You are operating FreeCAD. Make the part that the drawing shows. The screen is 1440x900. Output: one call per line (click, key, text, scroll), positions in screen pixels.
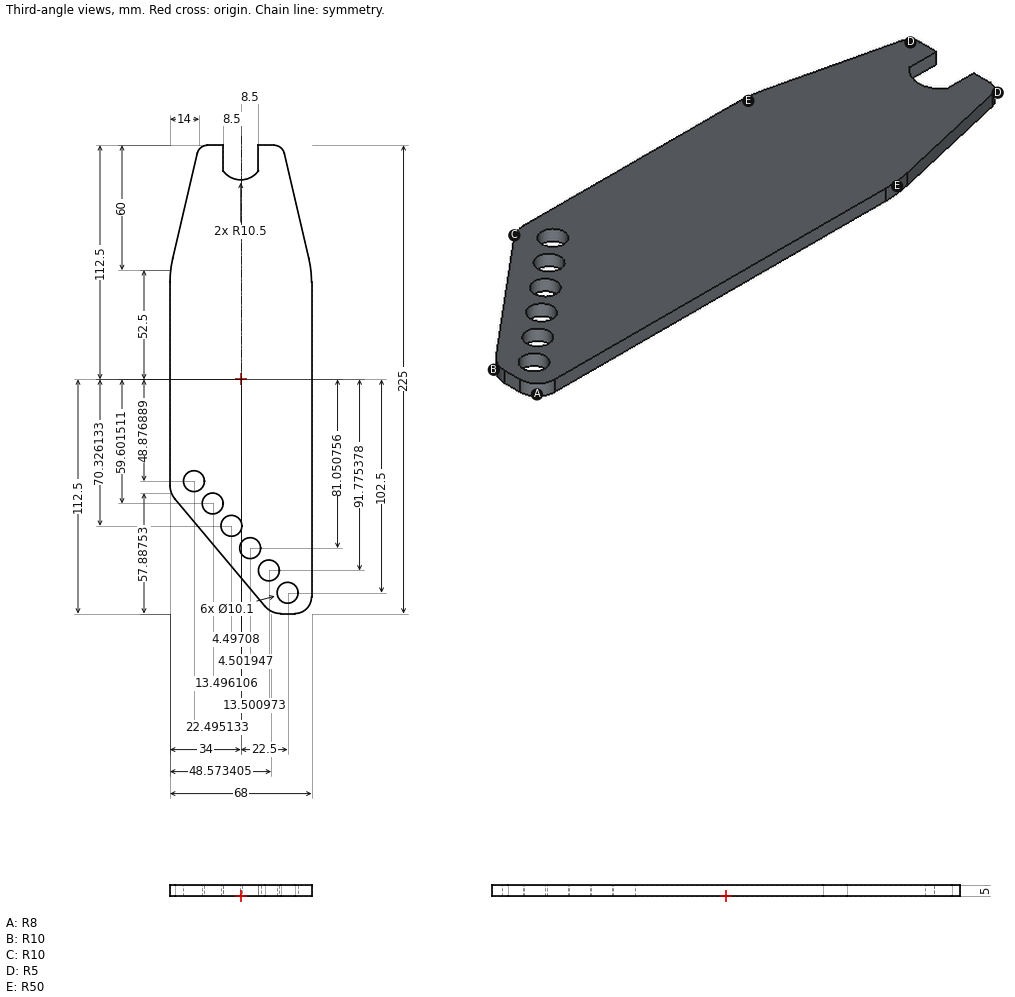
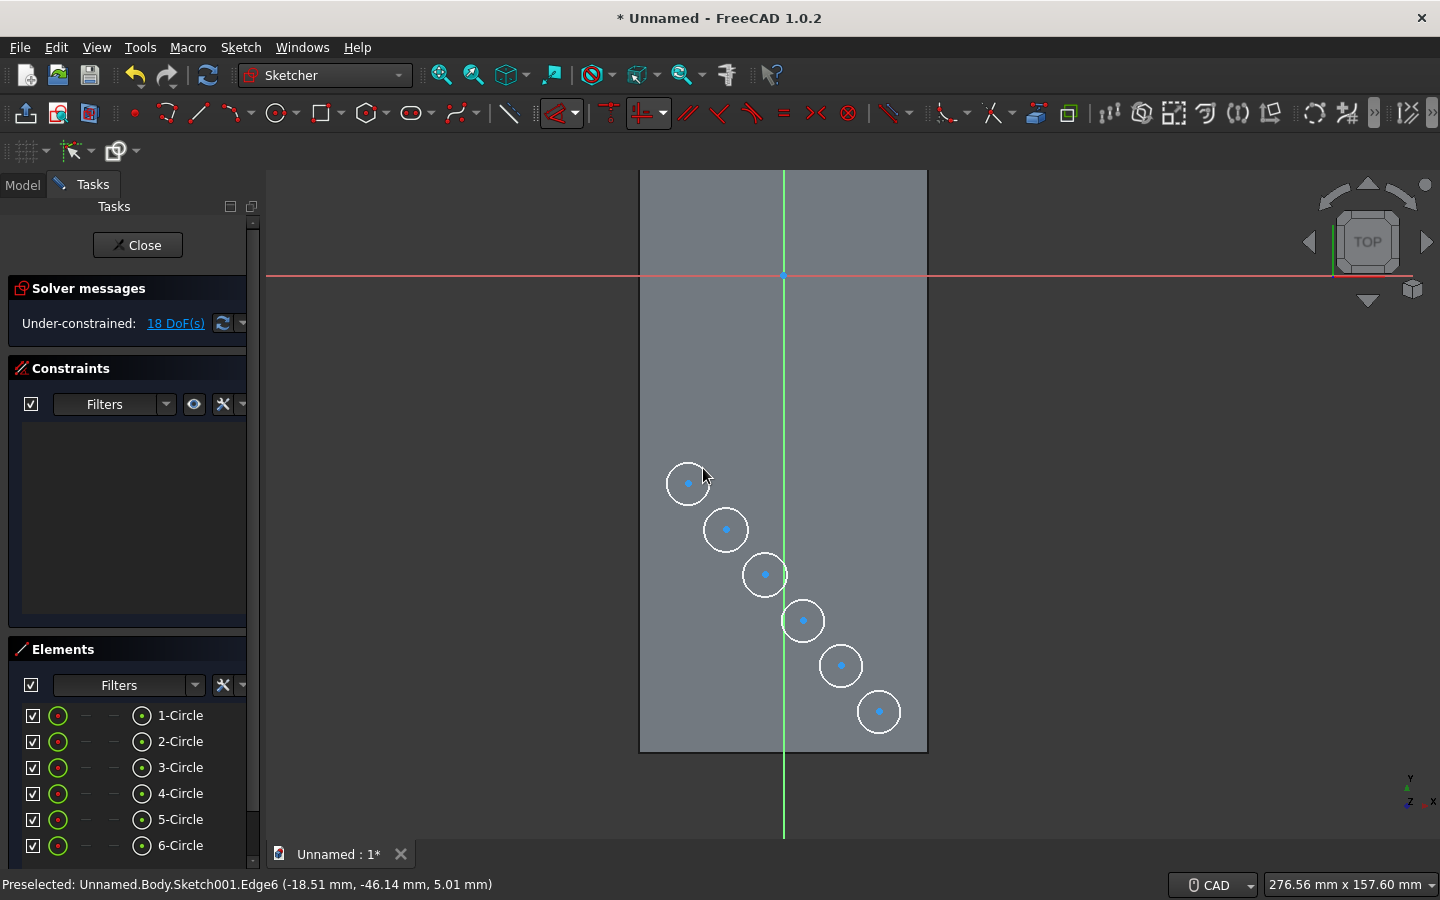
click(894, 697)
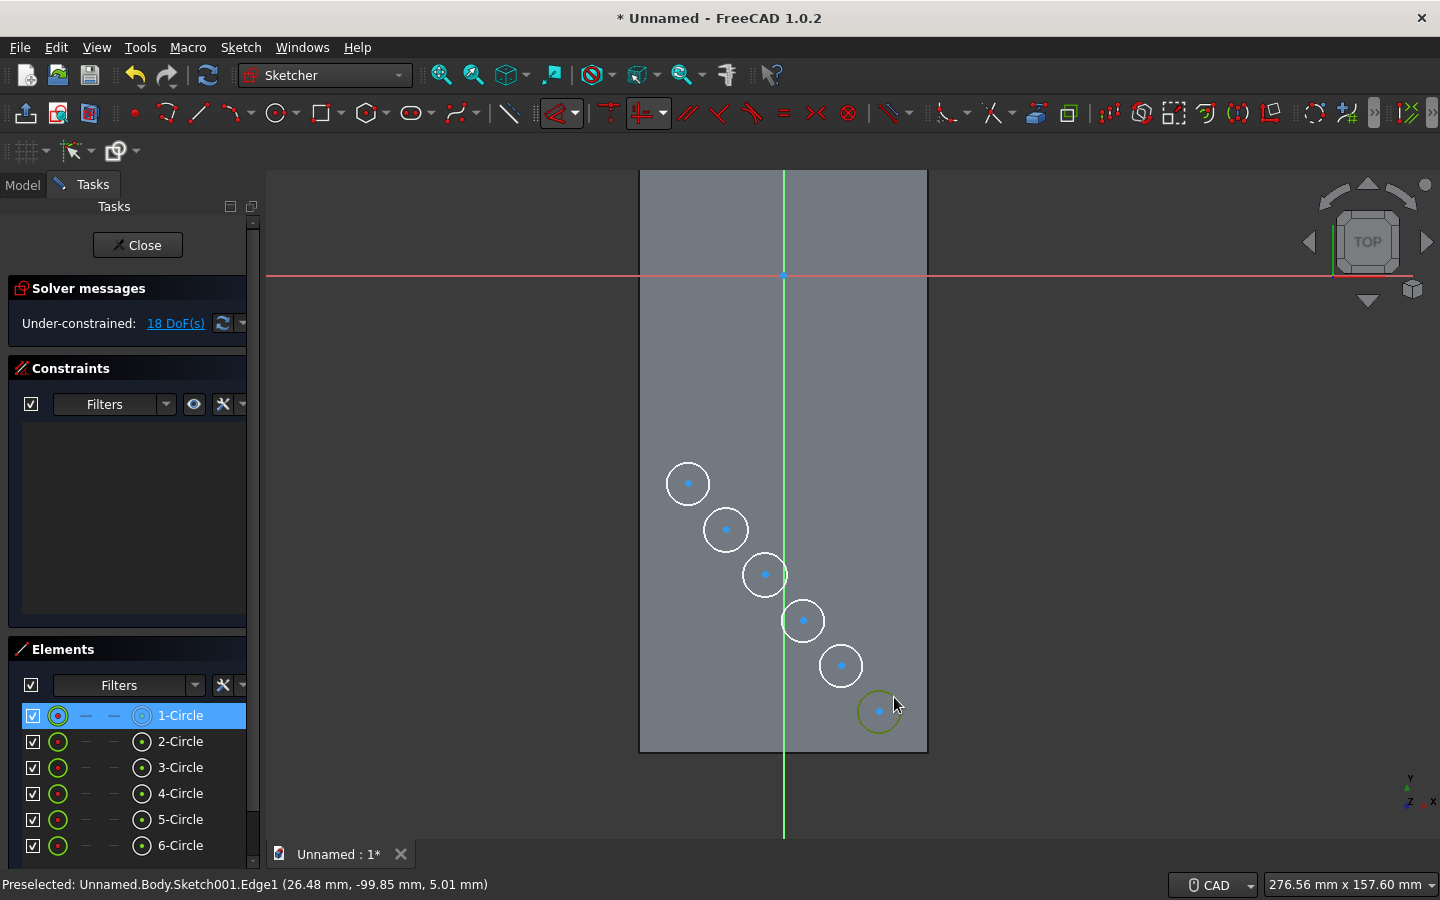
click(856, 651)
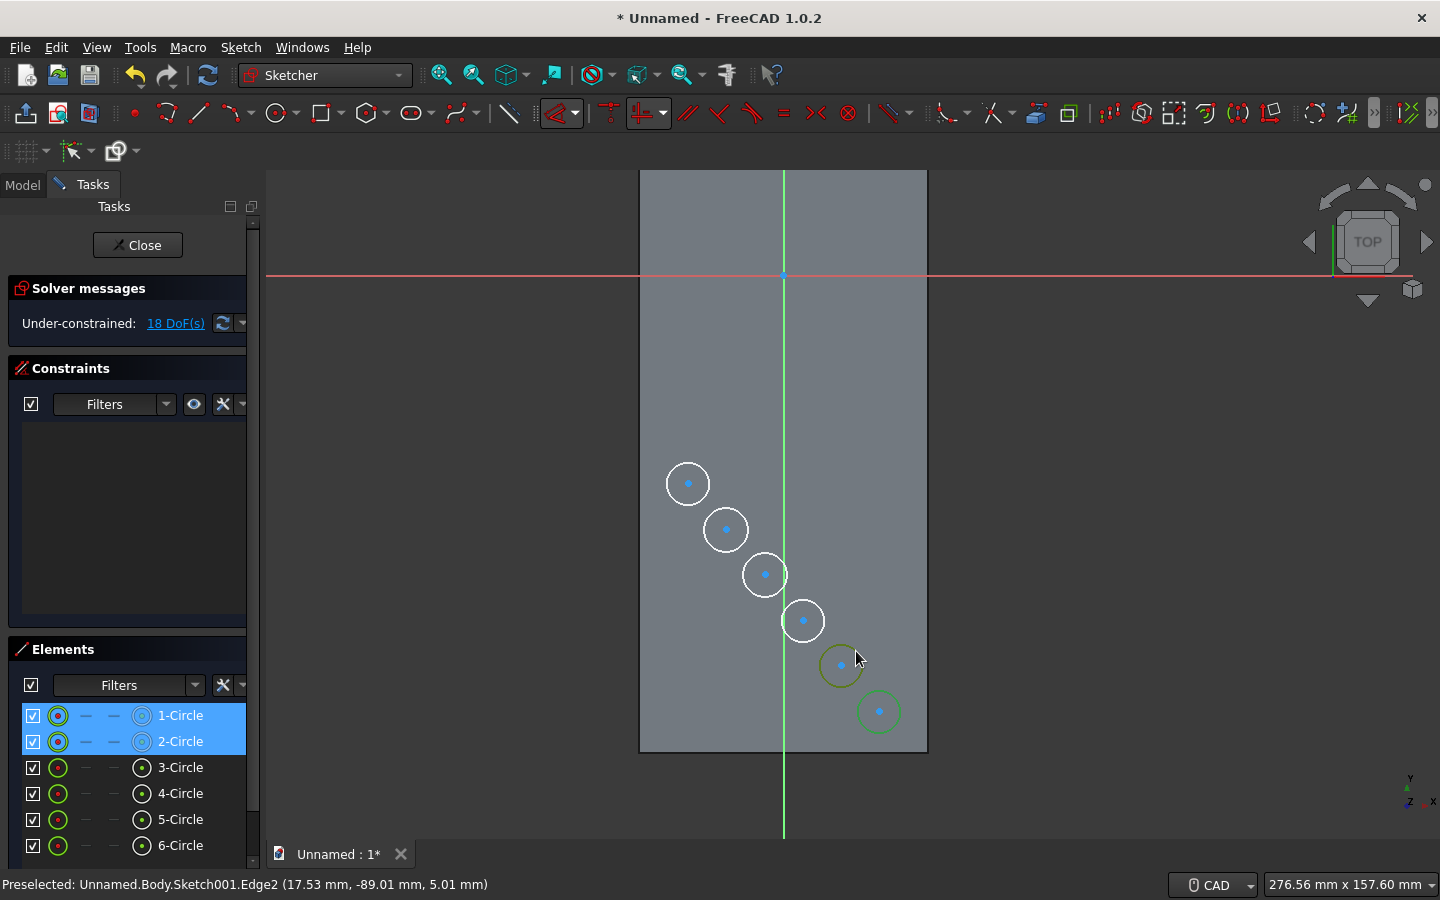
click(818, 606)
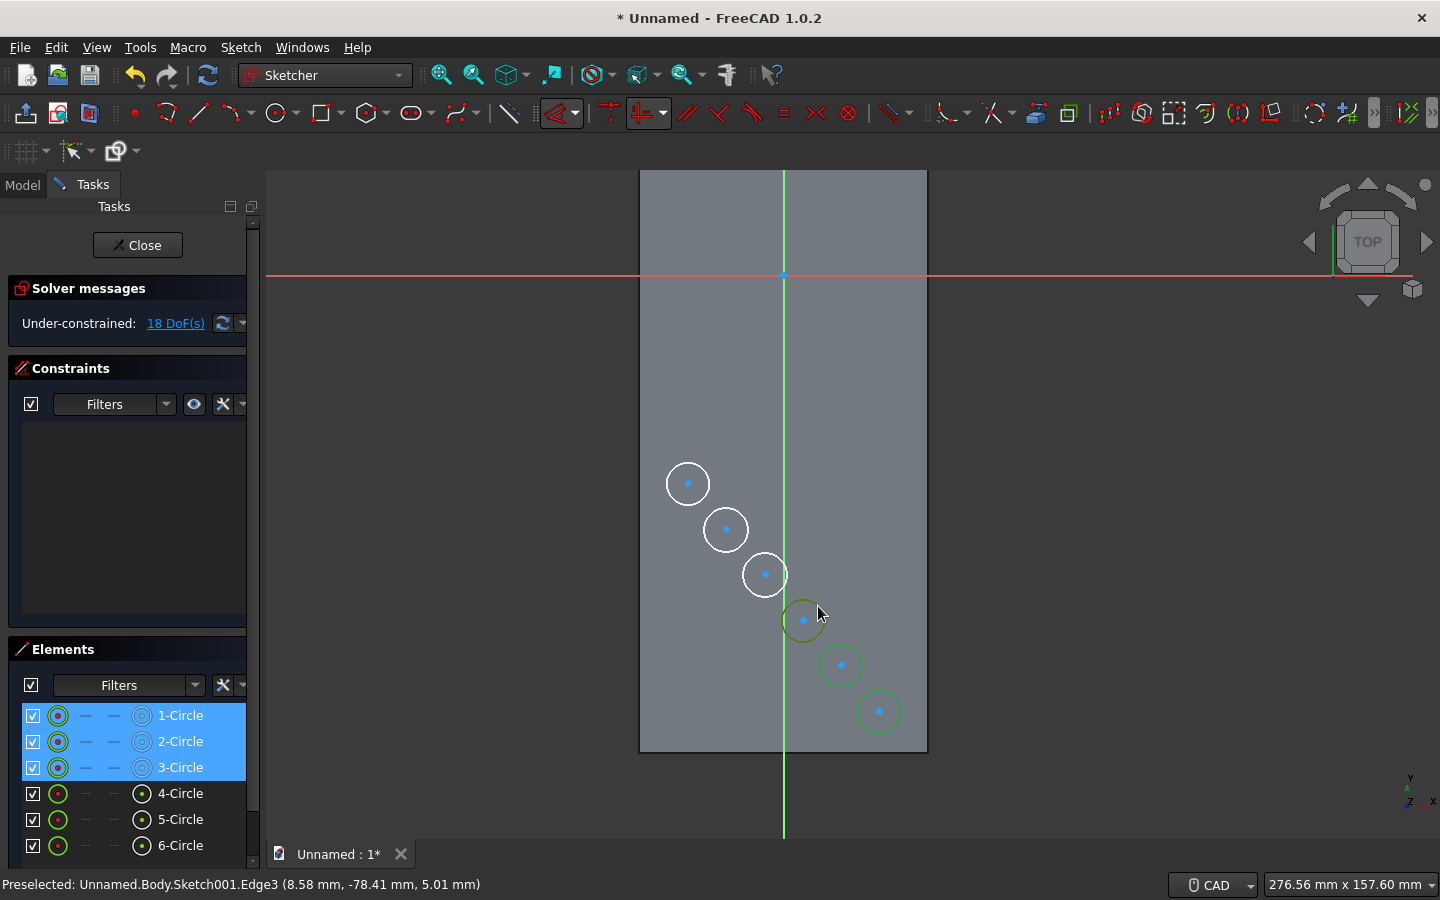
click(780, 559)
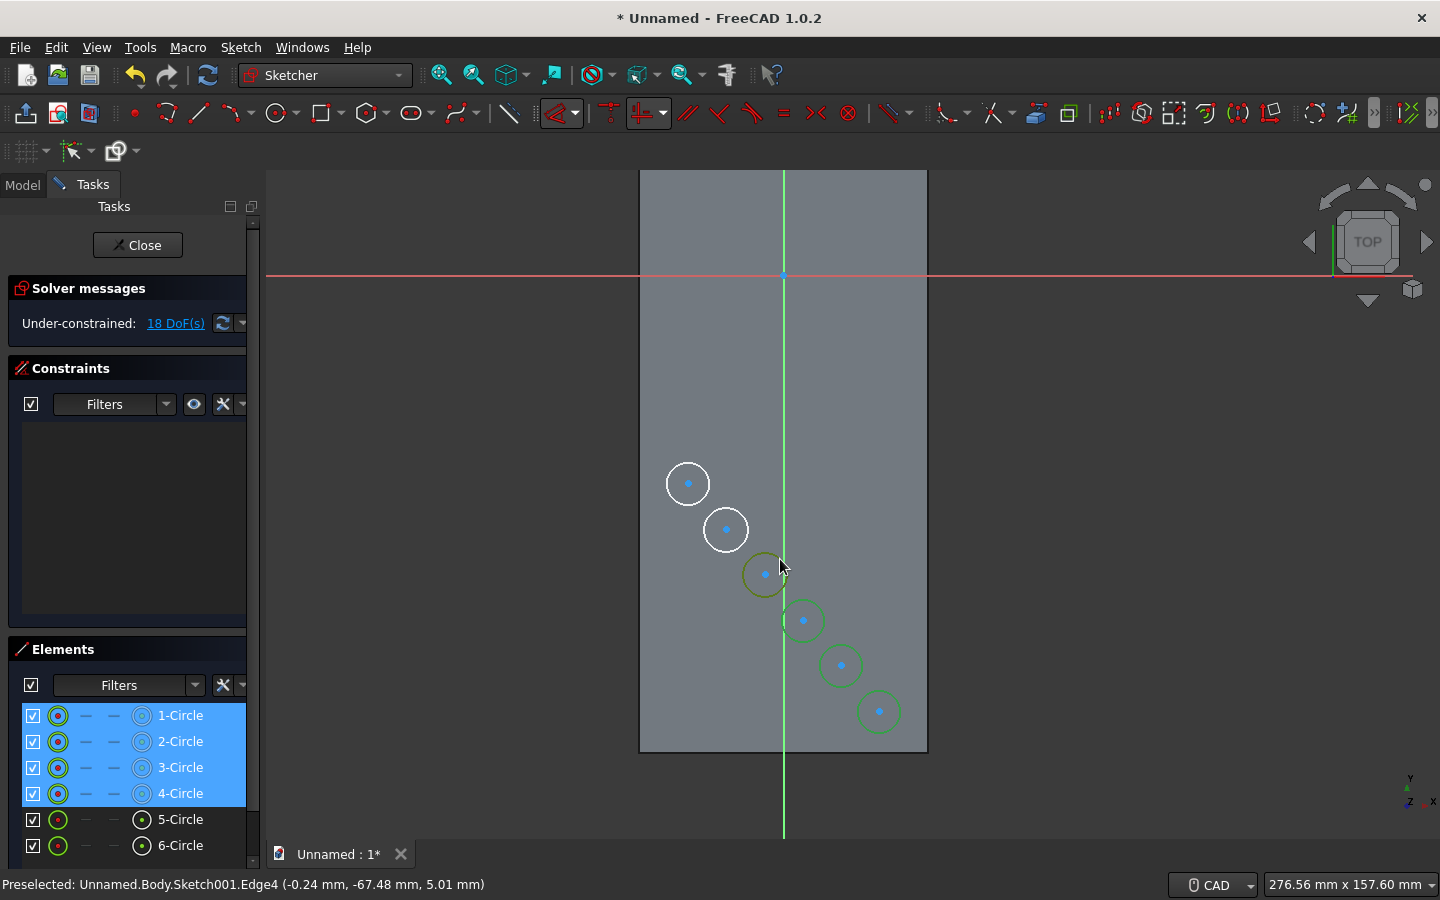
click(741, 514)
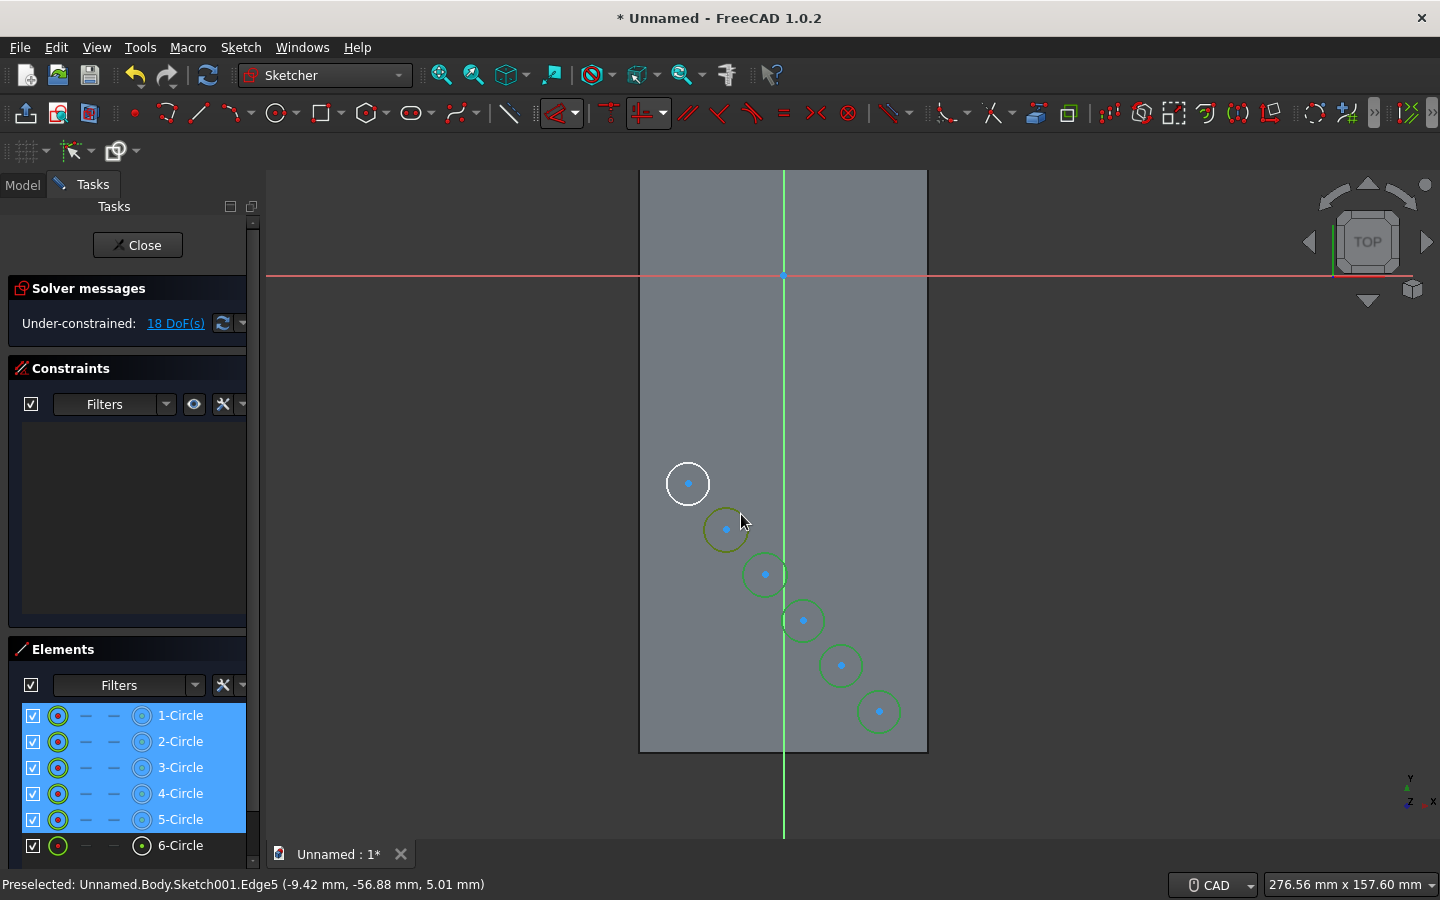
click(703, 469)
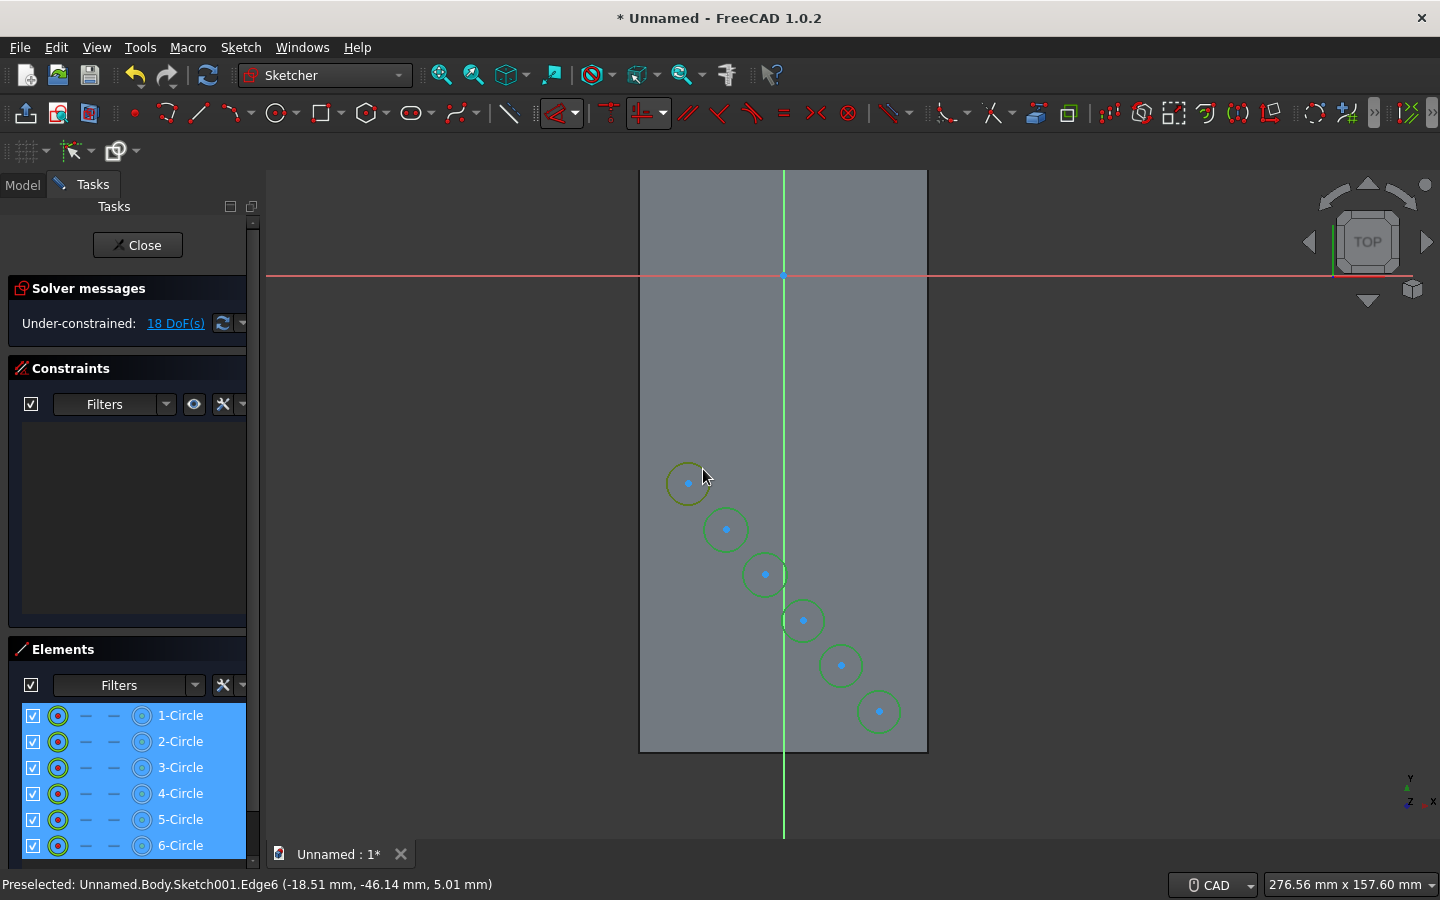
key(e)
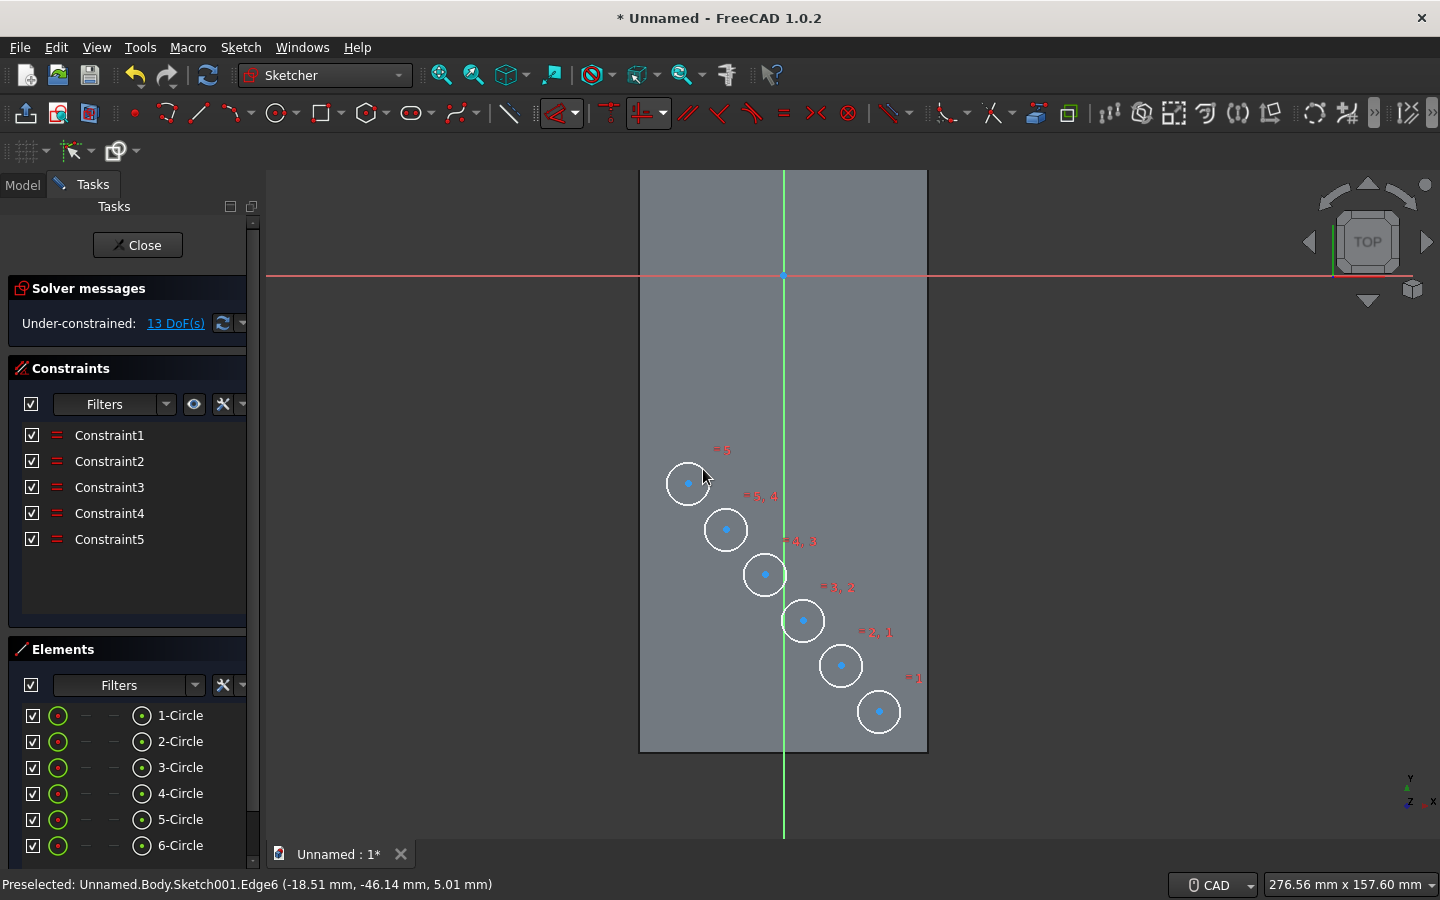
click(894, 697)